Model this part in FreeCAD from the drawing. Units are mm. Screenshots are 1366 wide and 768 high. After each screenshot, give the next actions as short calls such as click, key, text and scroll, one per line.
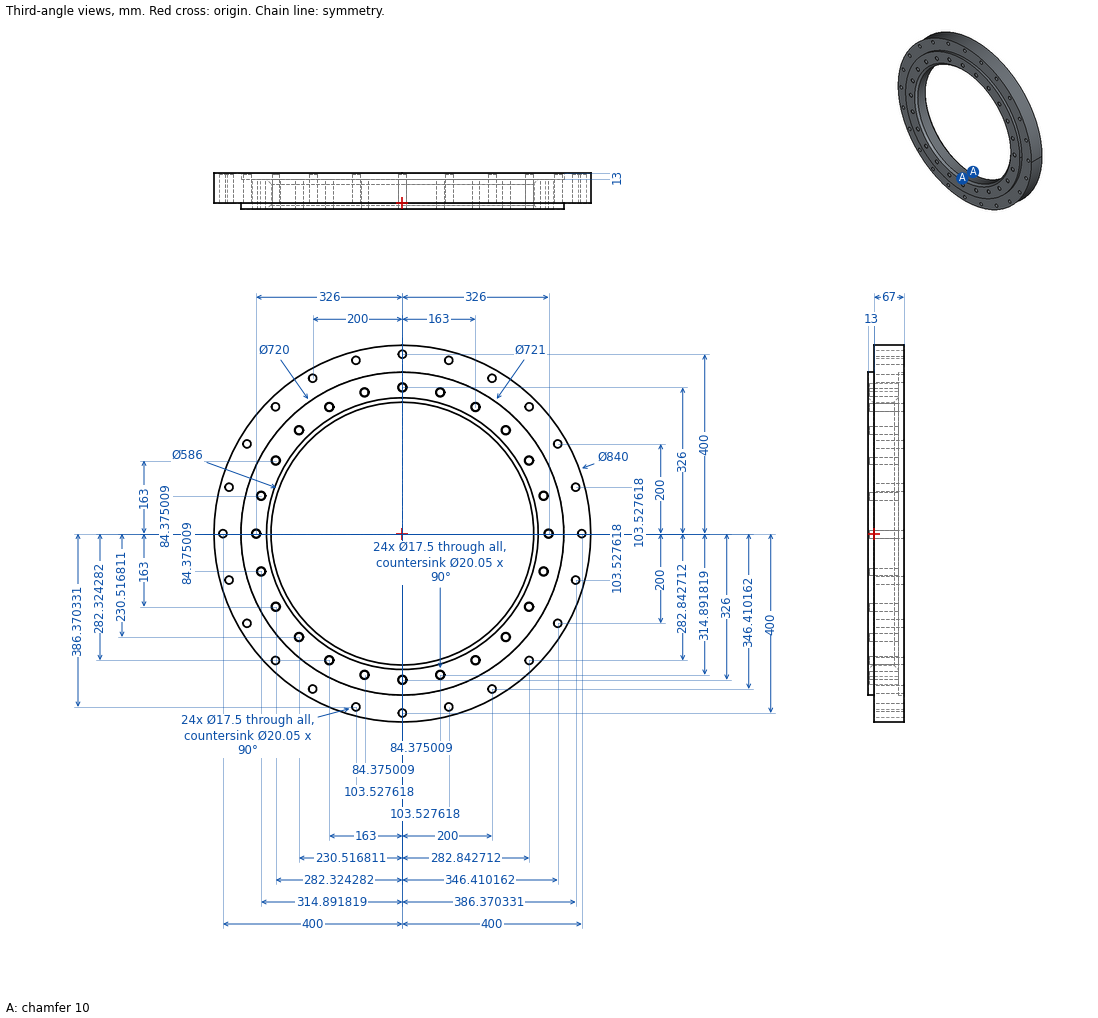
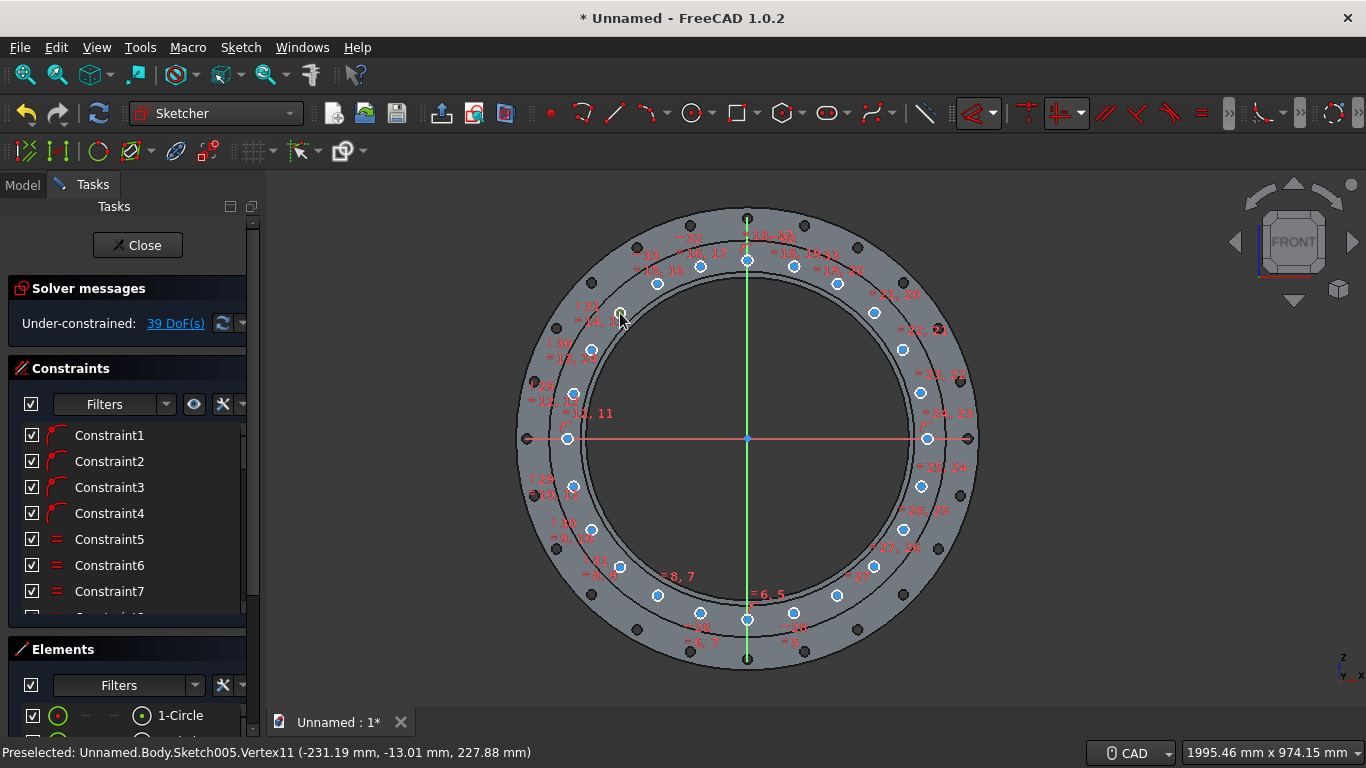
click(874, 313)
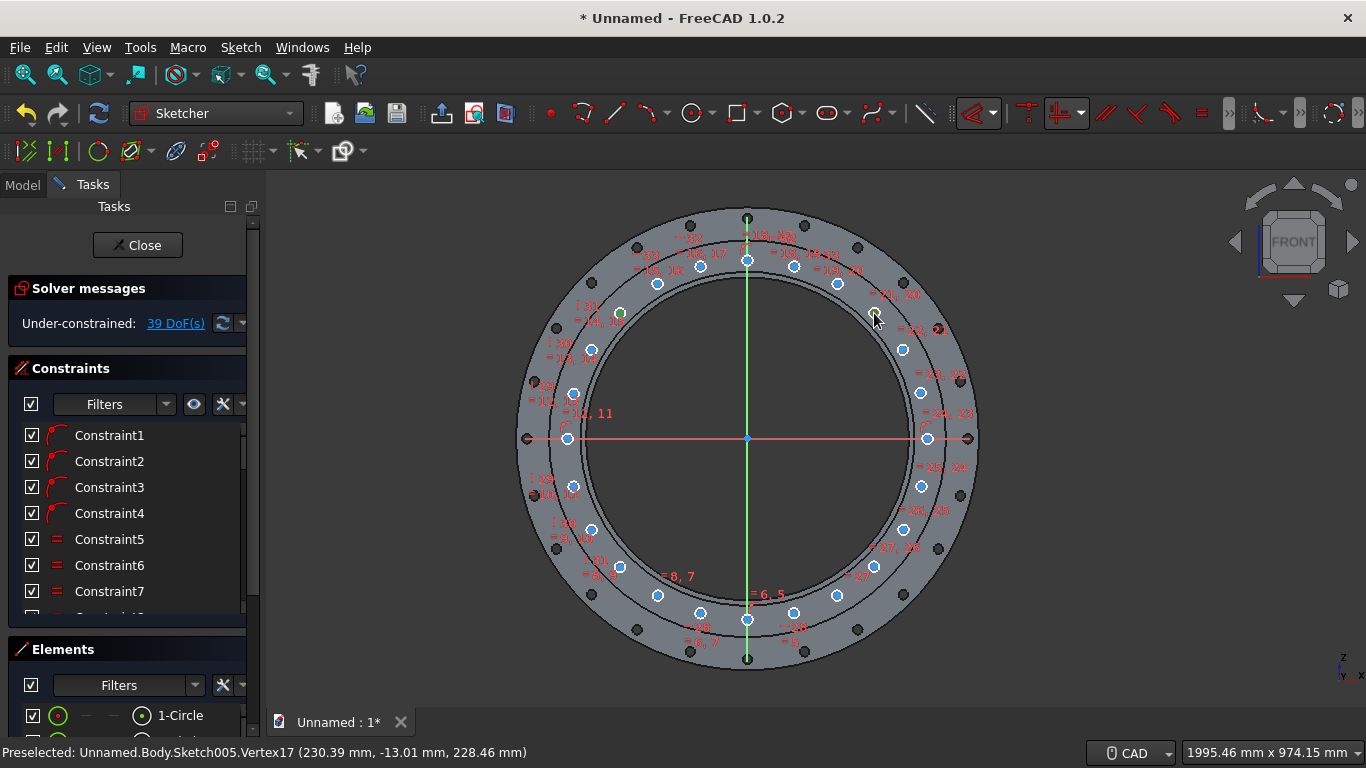
key(h)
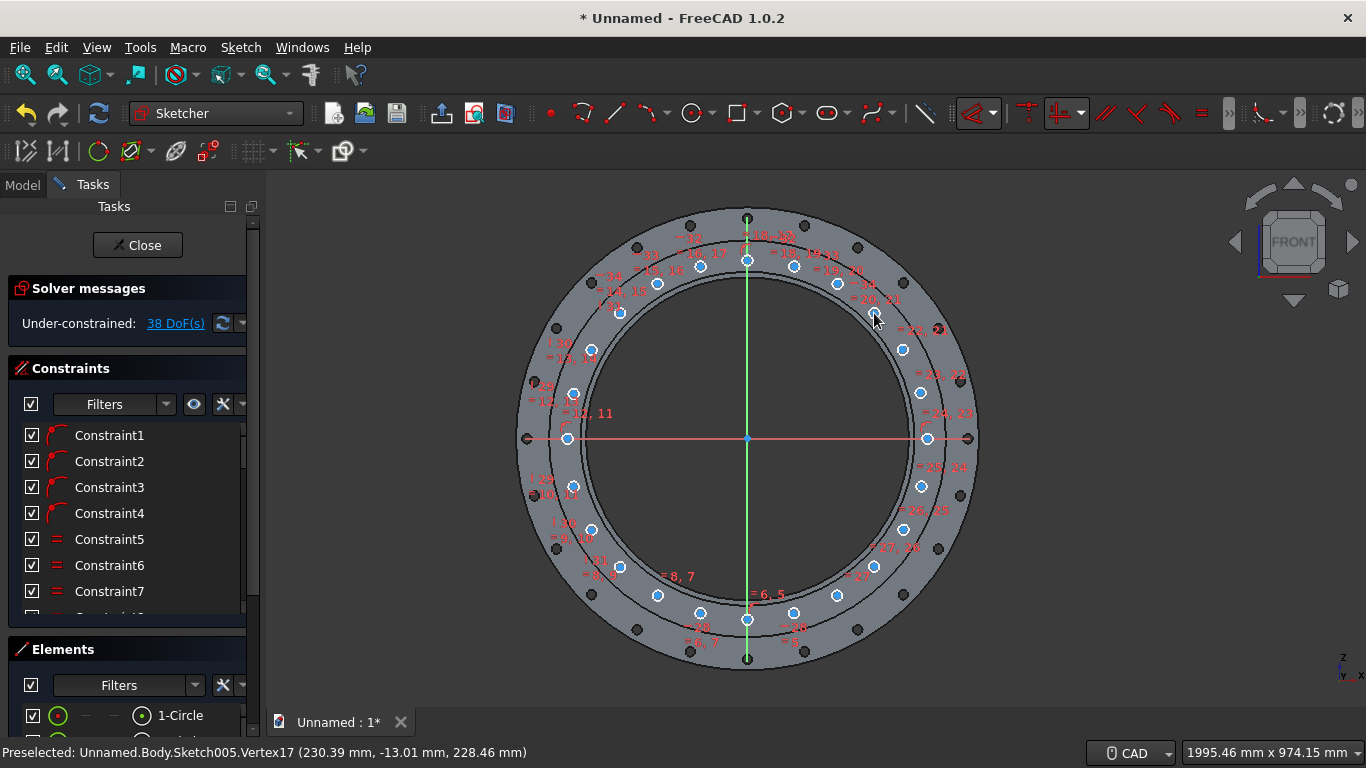
click(921, 393)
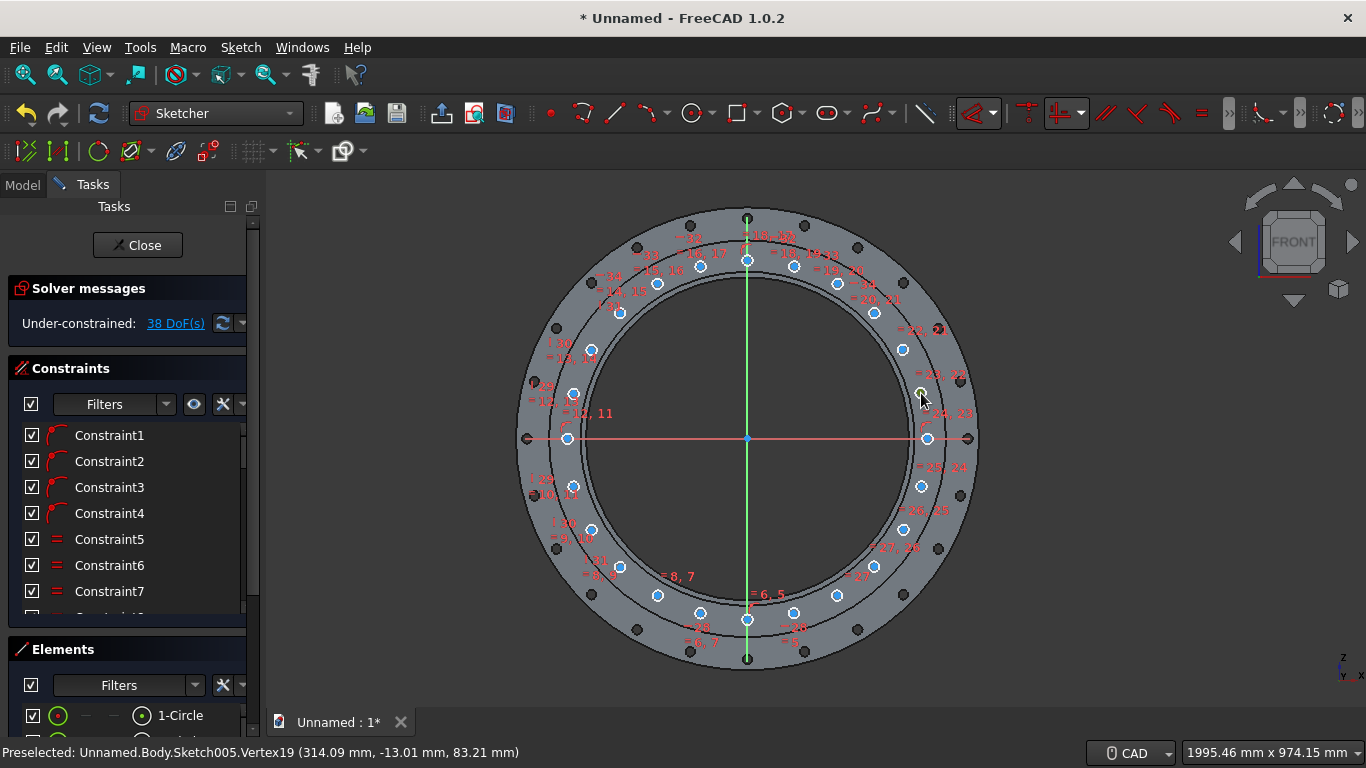
click(922, 487)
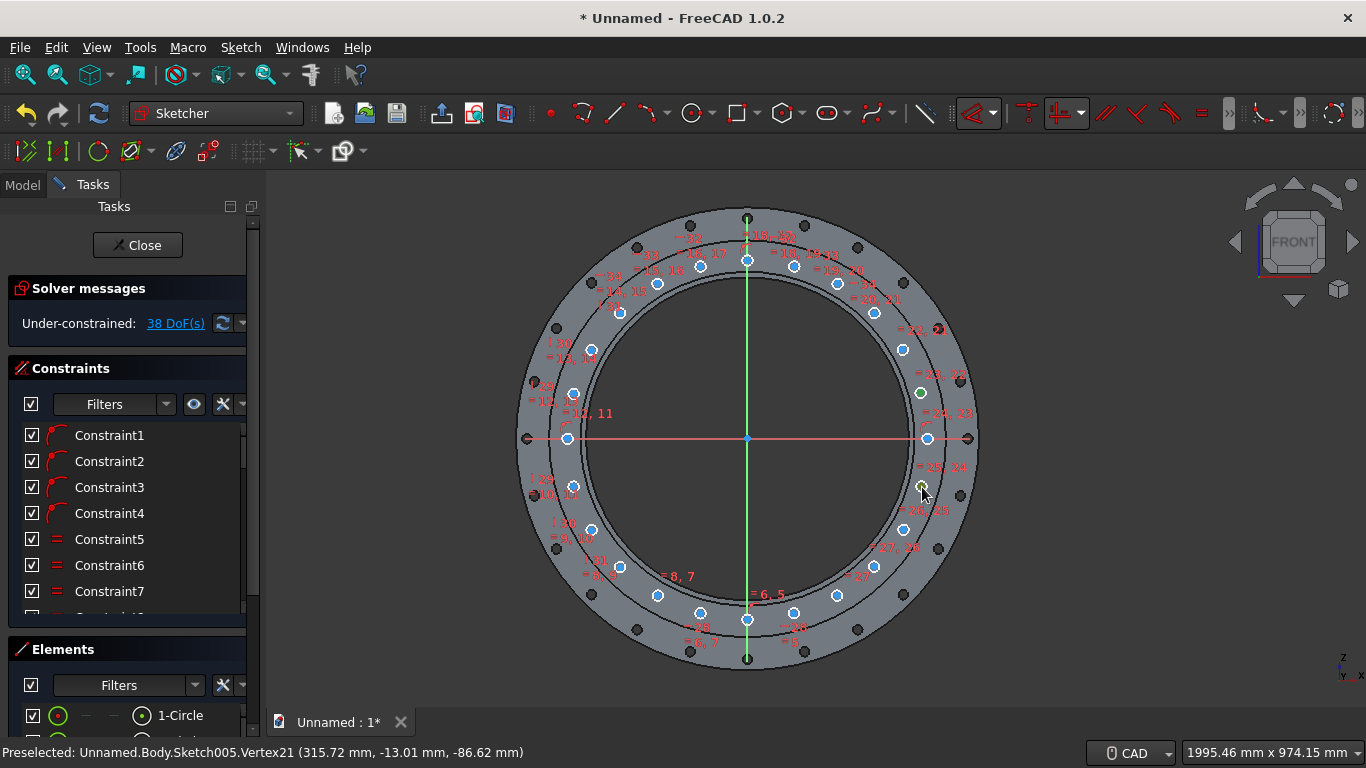
key(v)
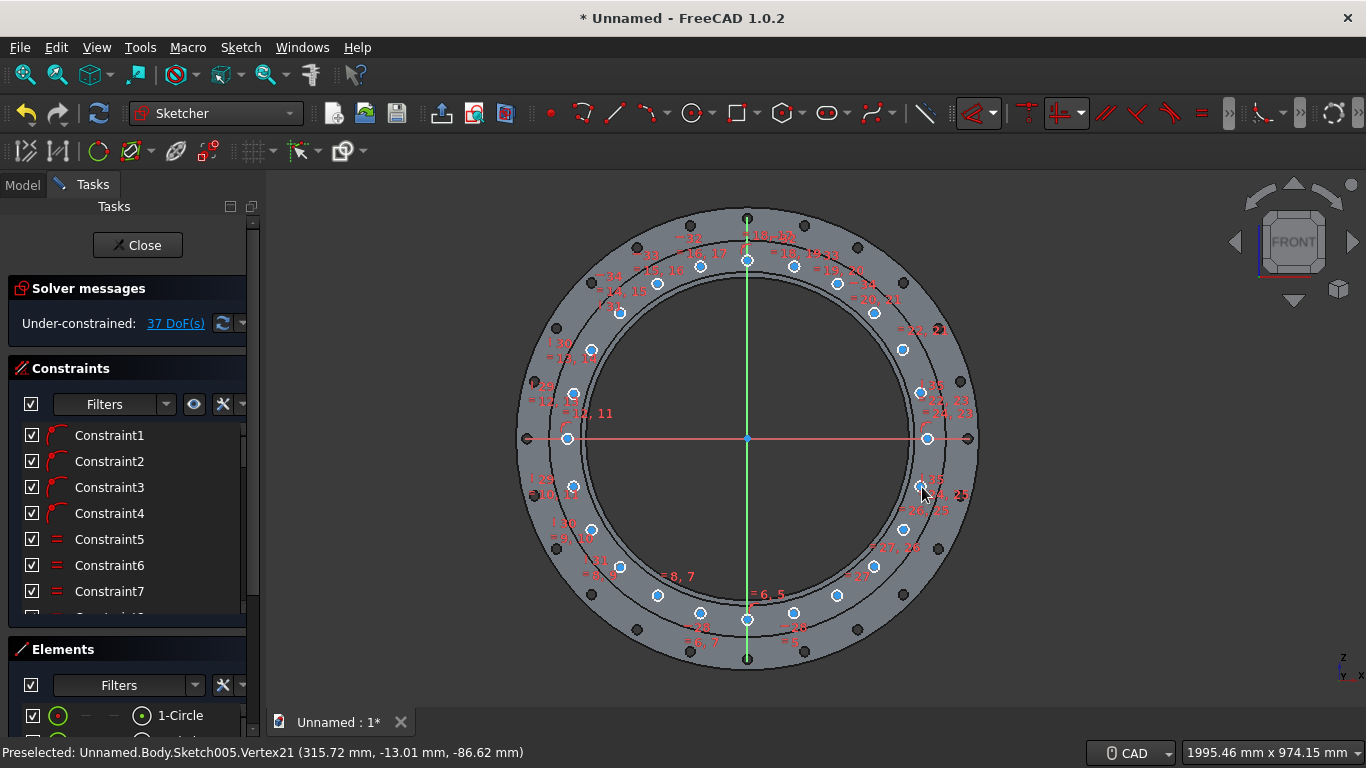
click(903, 350)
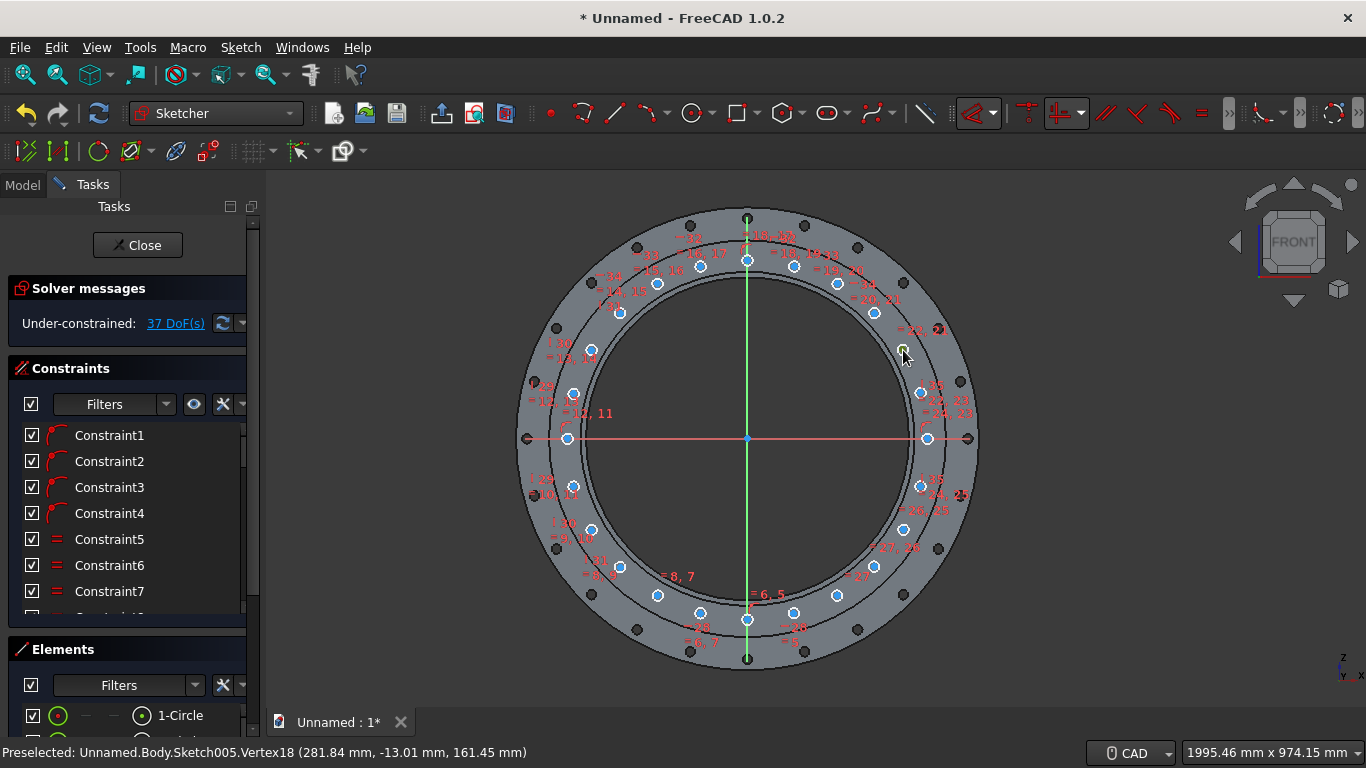
click(904, 530)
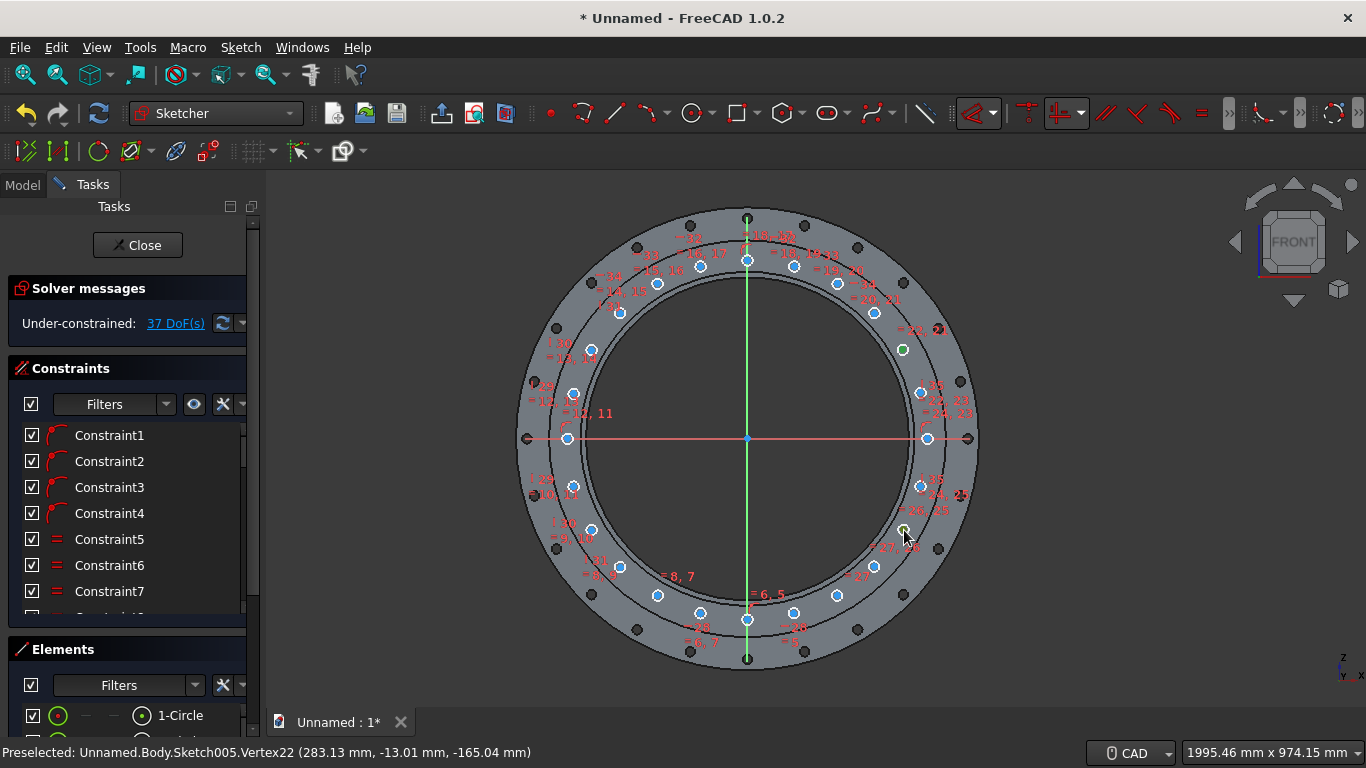
key(v)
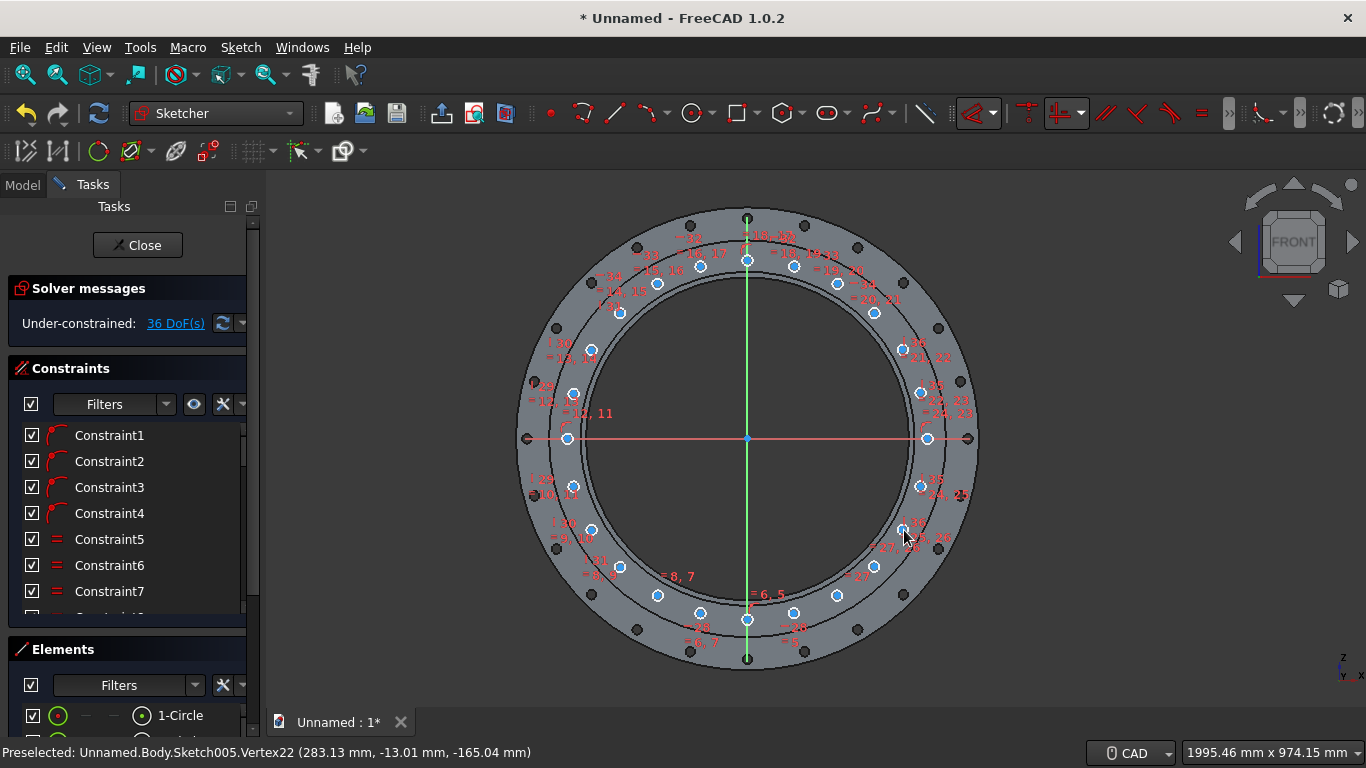
click(658, 596)